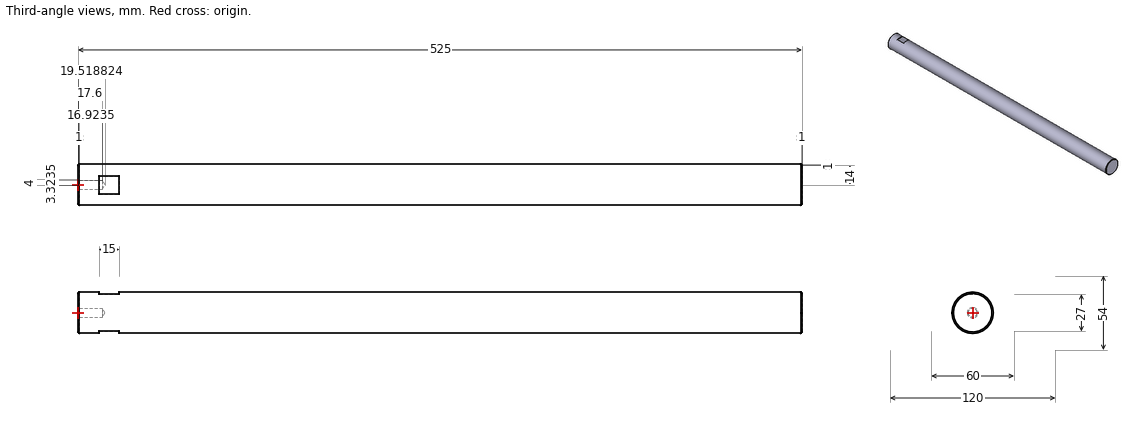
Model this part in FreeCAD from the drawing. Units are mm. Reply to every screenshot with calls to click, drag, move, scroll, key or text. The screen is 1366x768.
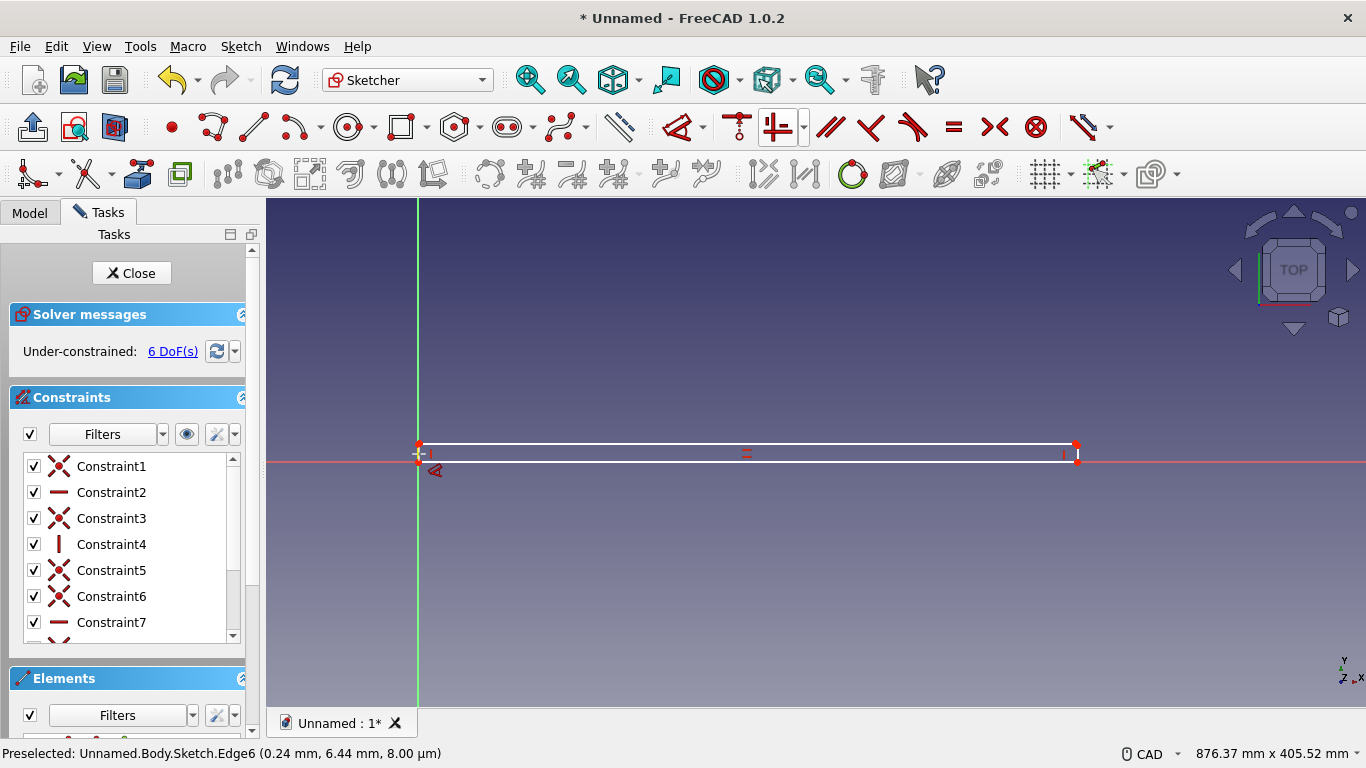
scroll(1078, 456, up, 5)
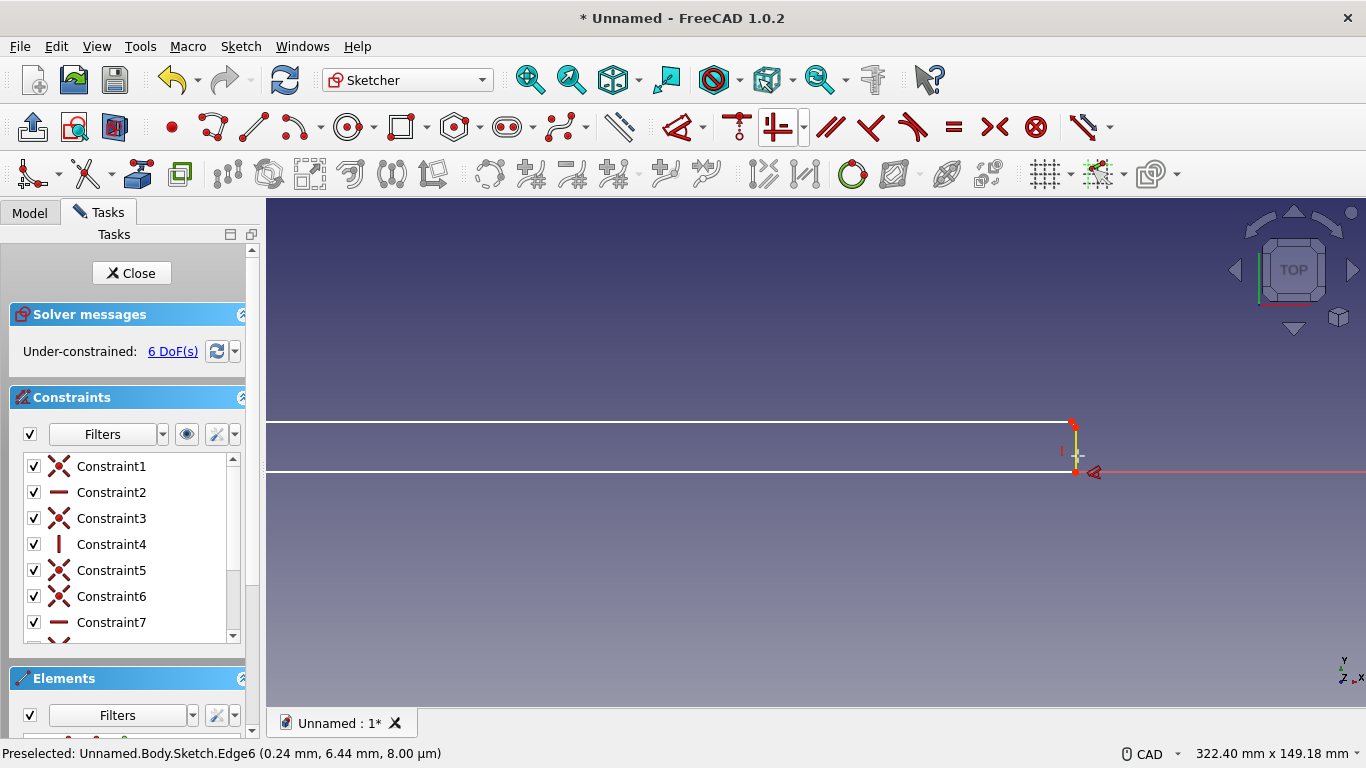
click(1076, 455)
click(1110, 450)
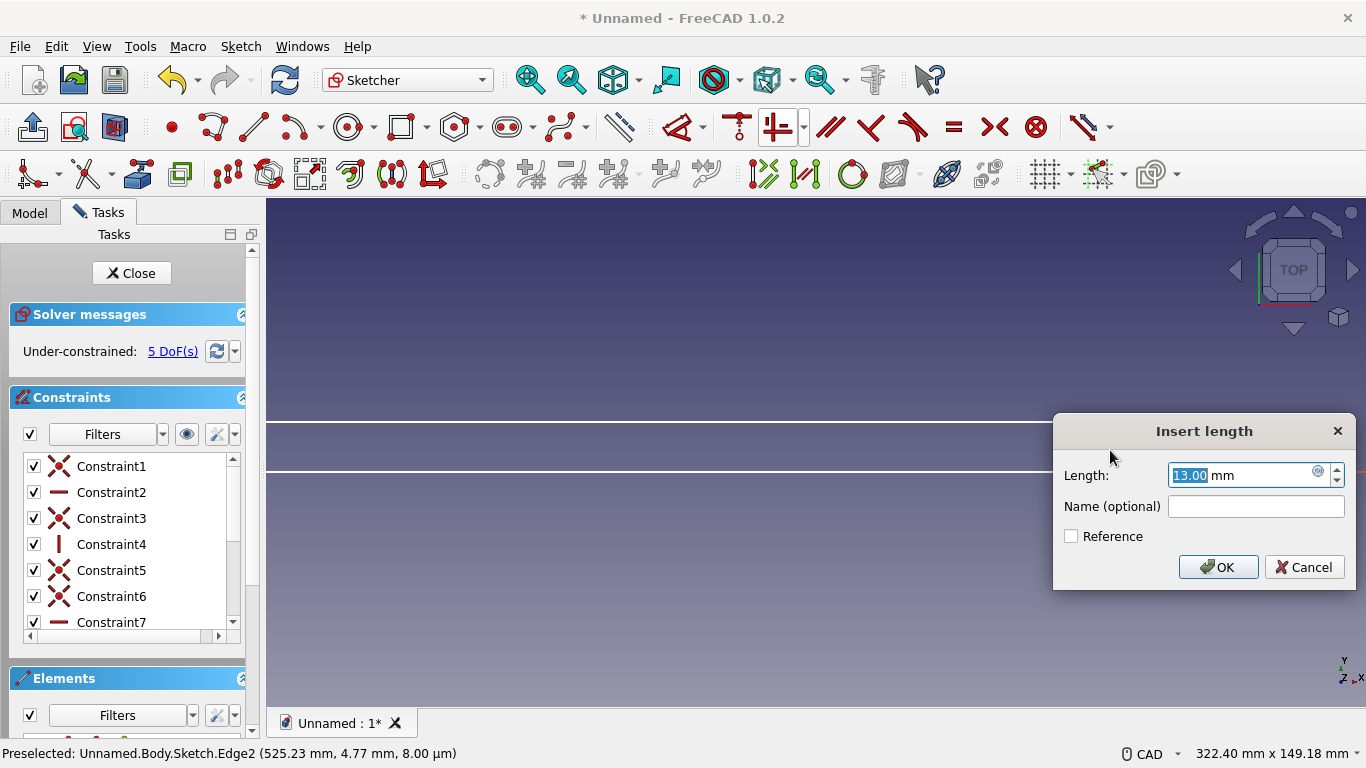
text(14)
key(Return)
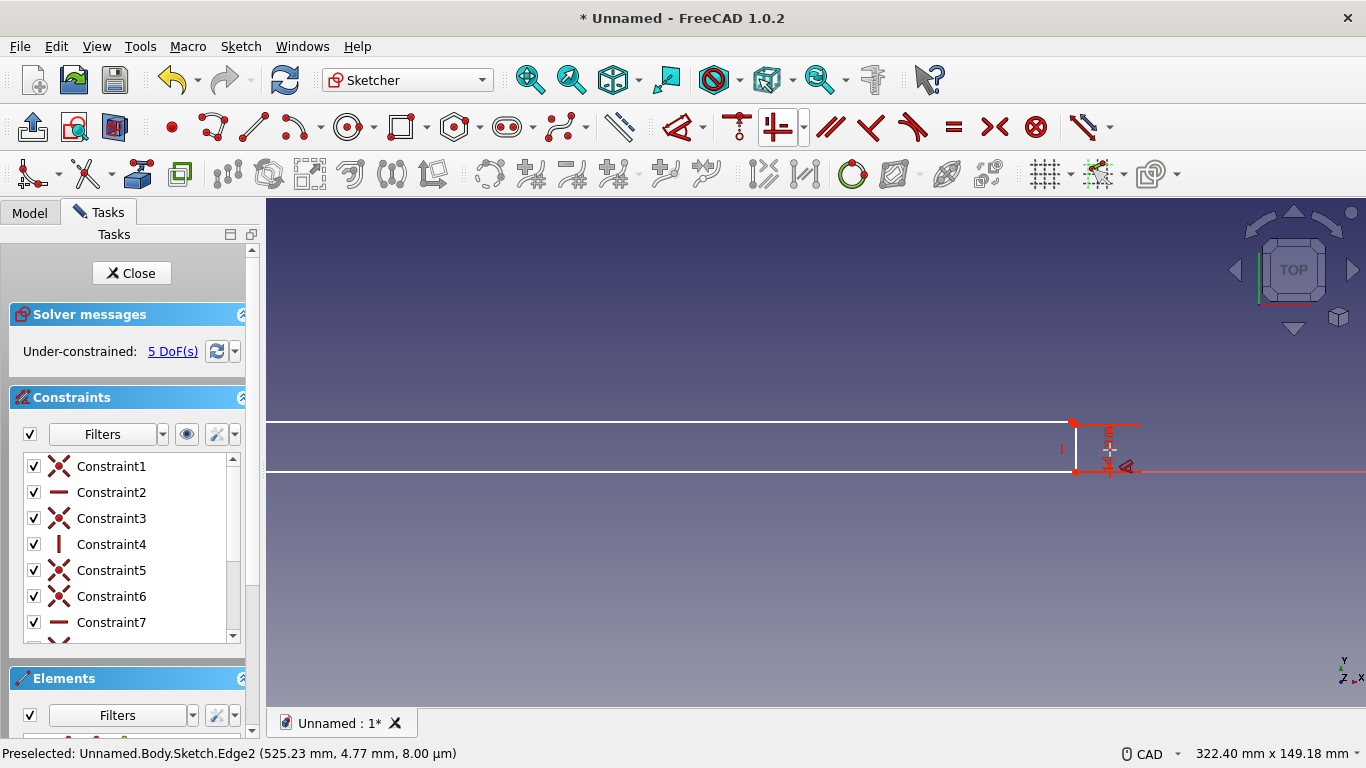
scroll(1078, 456, down, 5)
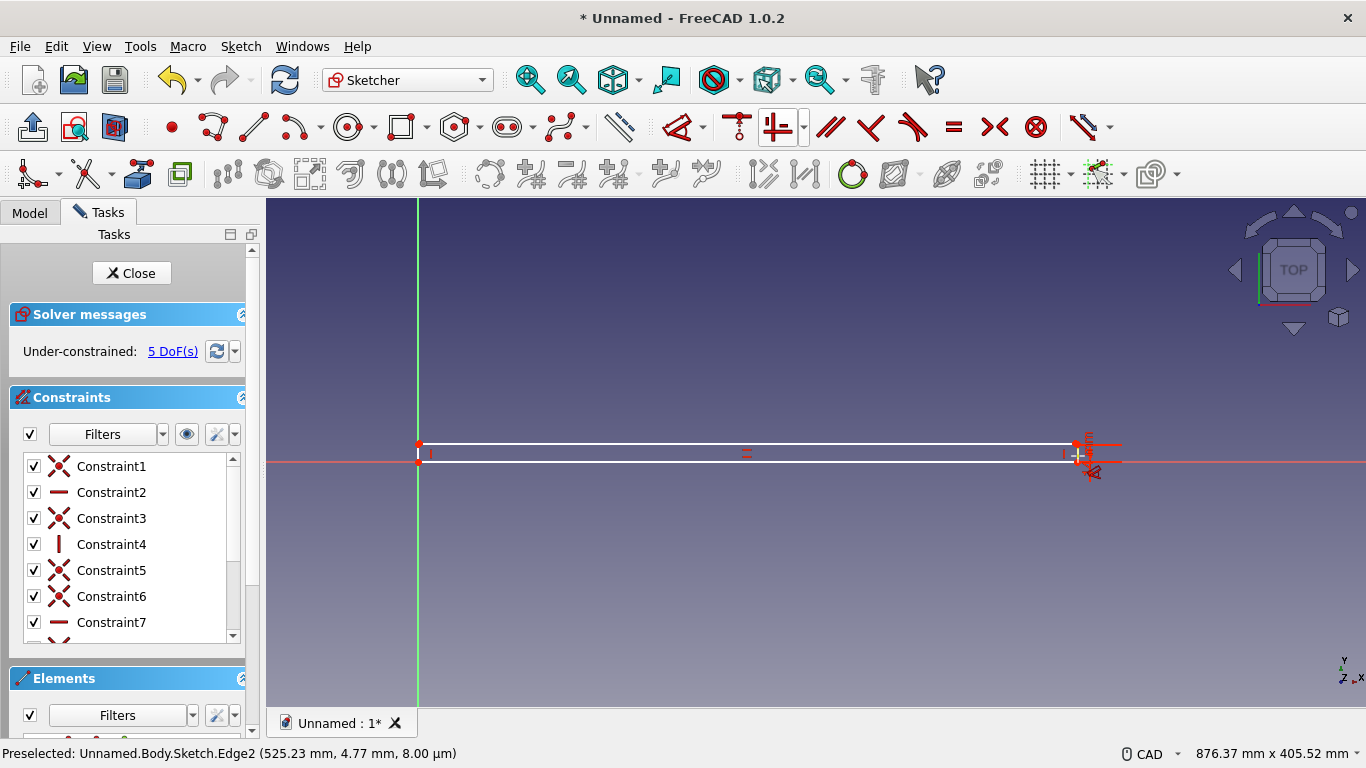
scroll(418, 450, up, 5)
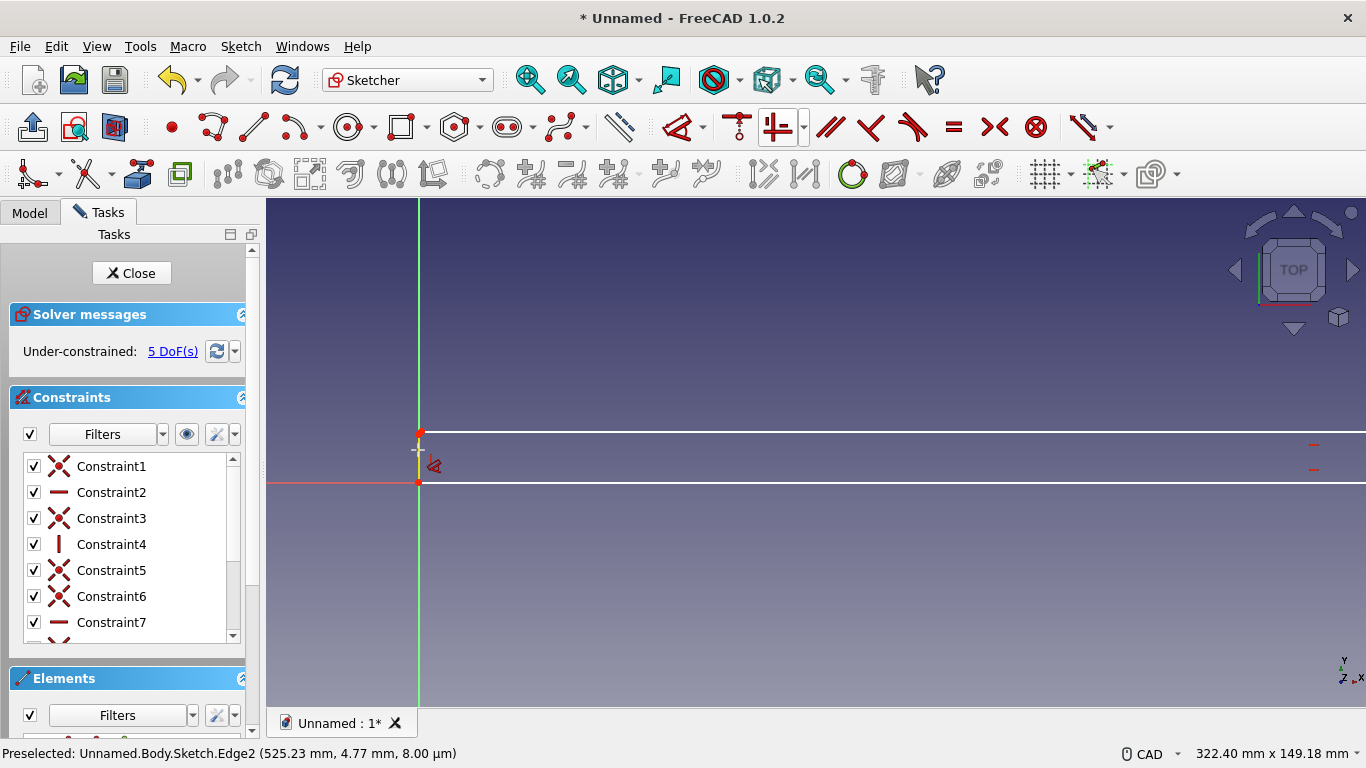
click(419, 449)
click(385, 459)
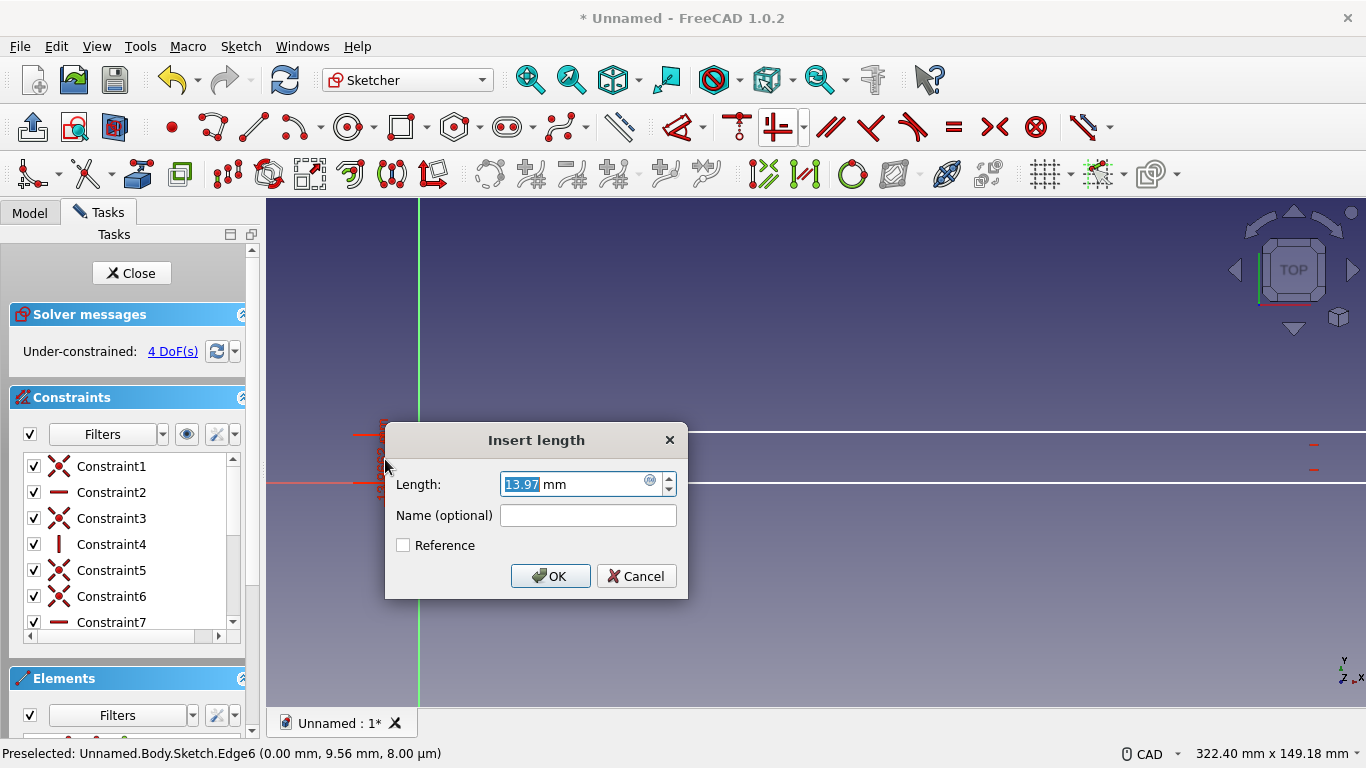
text(14)
key(Return)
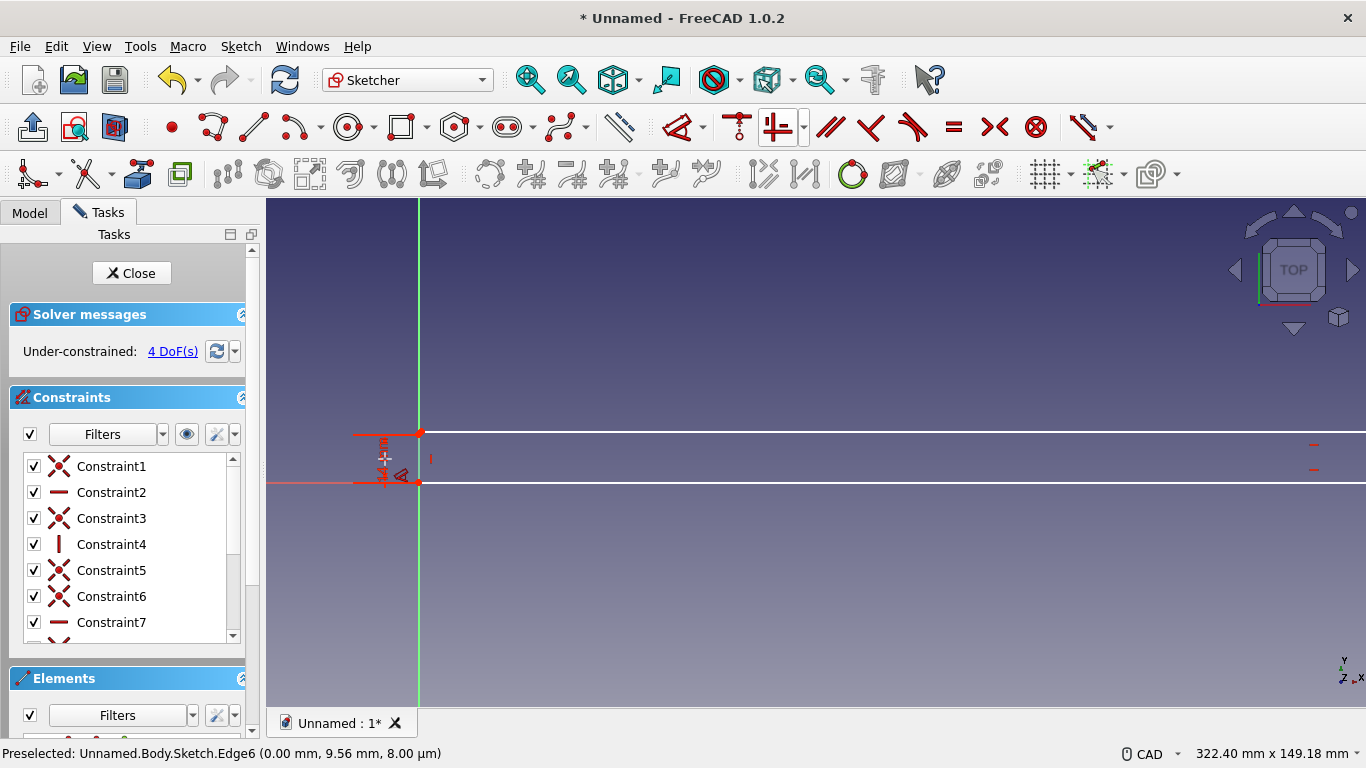
scroll(422, 432, up, 13)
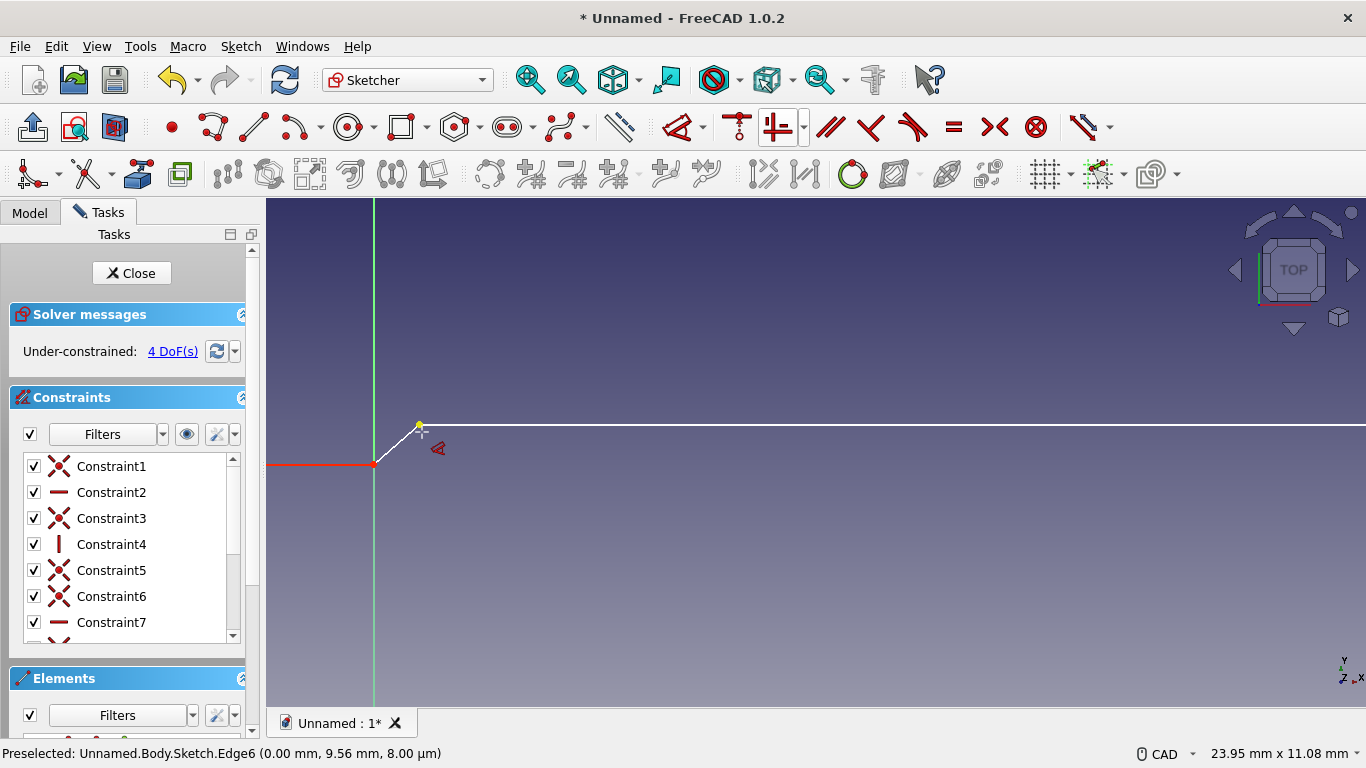
click(419, 425)
click(397, 391)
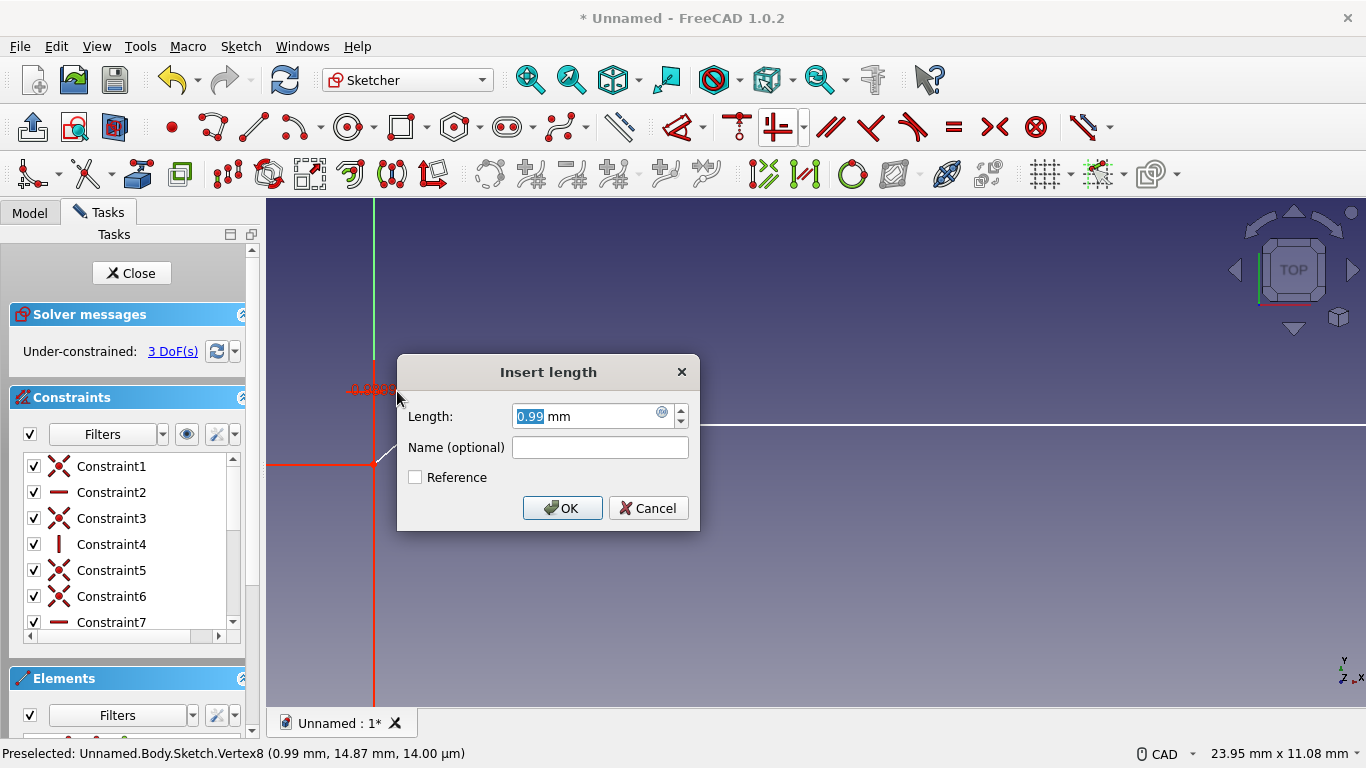
text(1)
key(Return)